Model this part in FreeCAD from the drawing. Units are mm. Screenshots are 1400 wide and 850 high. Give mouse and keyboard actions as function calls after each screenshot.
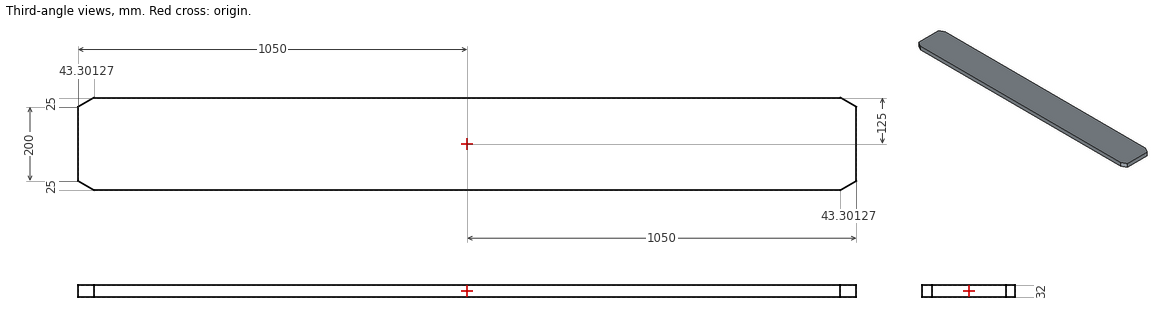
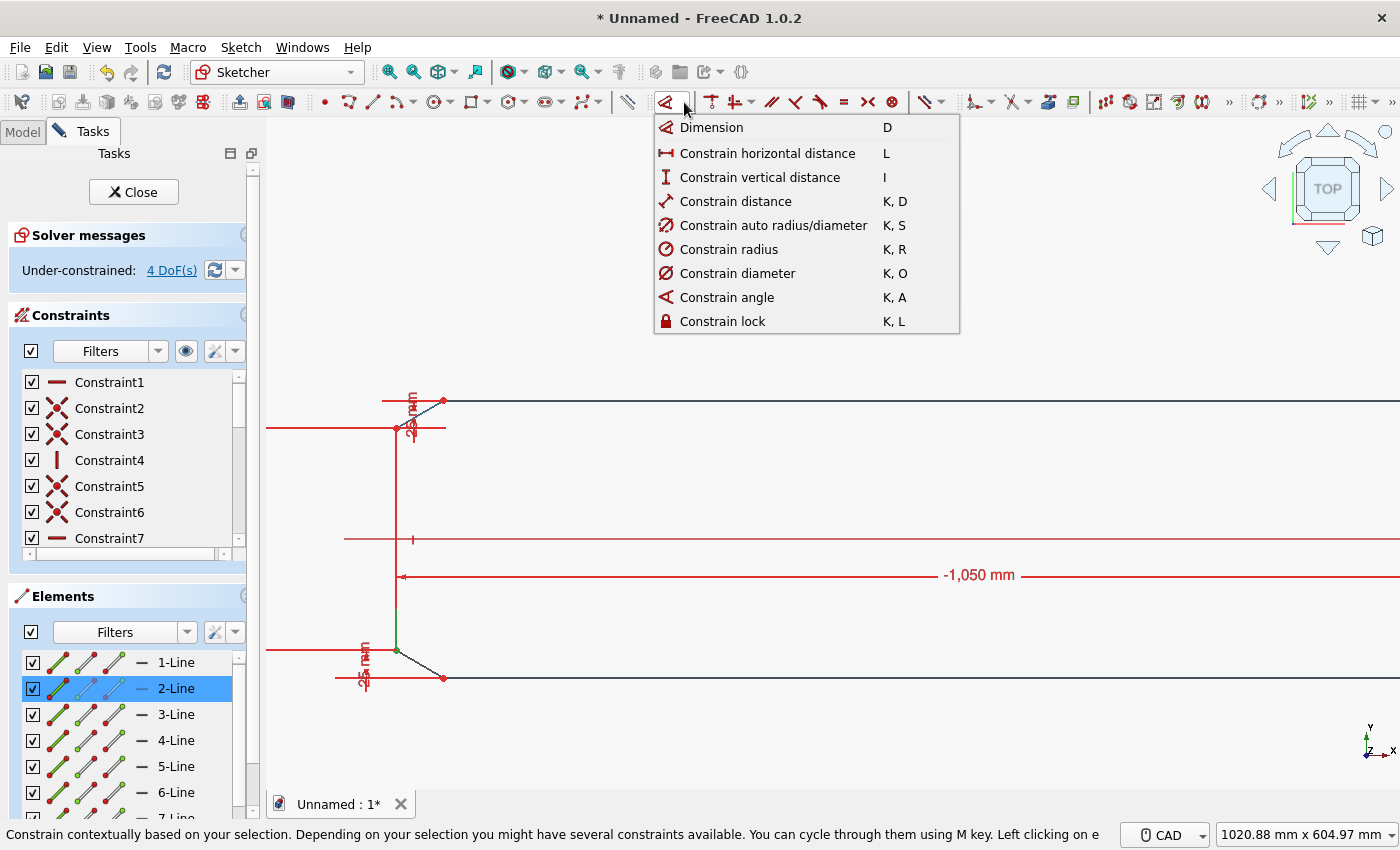
click(807, 153)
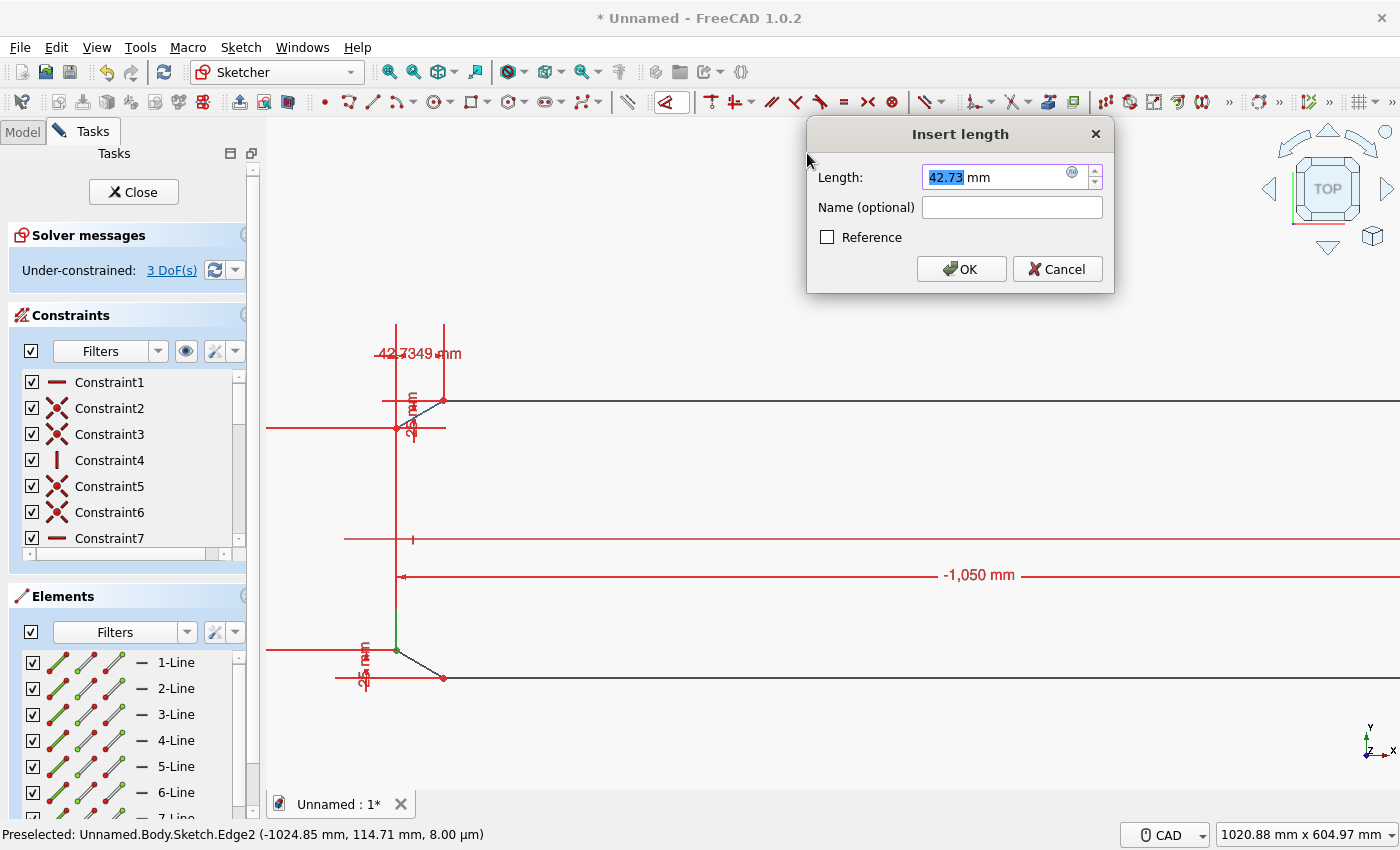
text(43.30127)
key(Return)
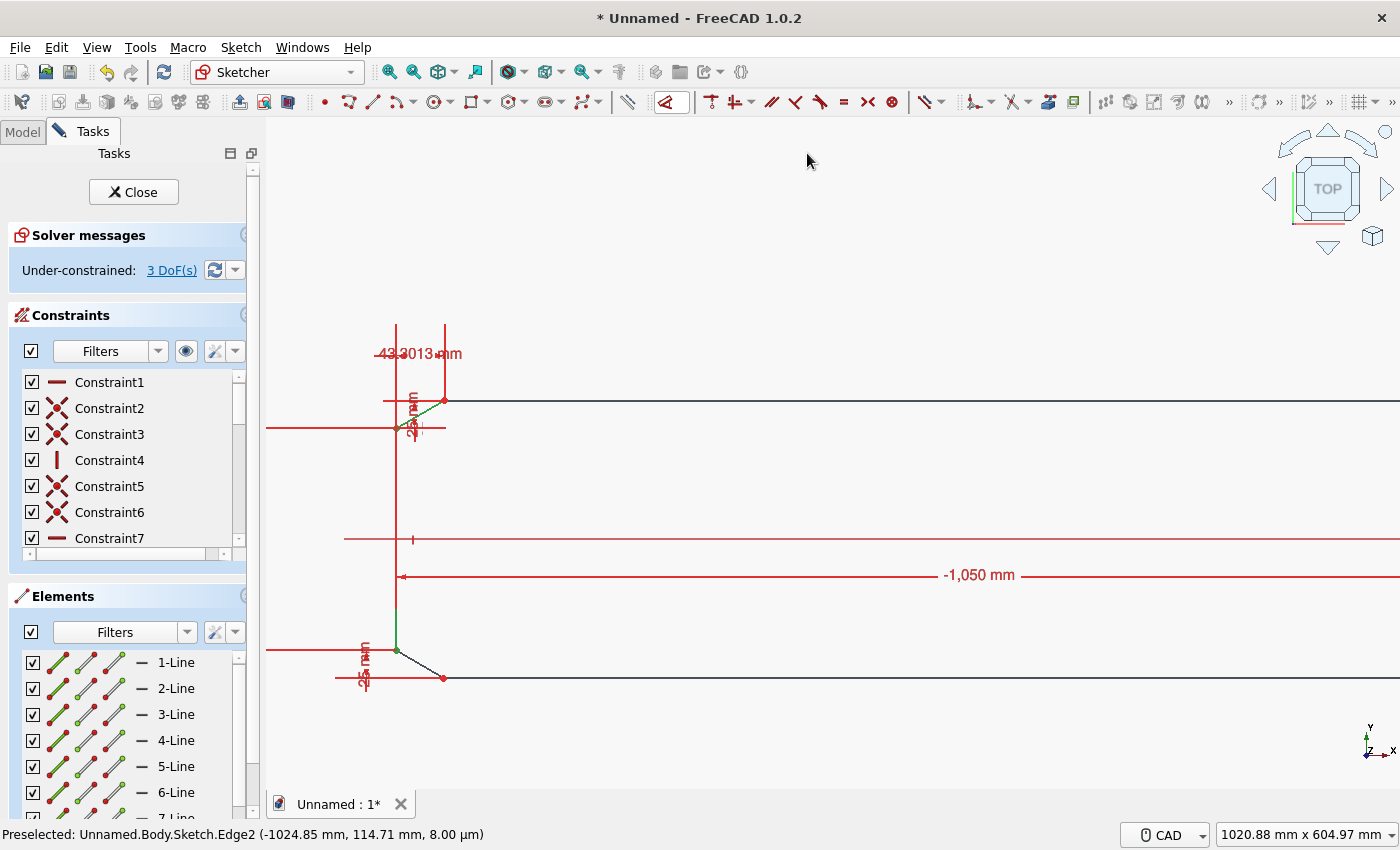
click(411, 659)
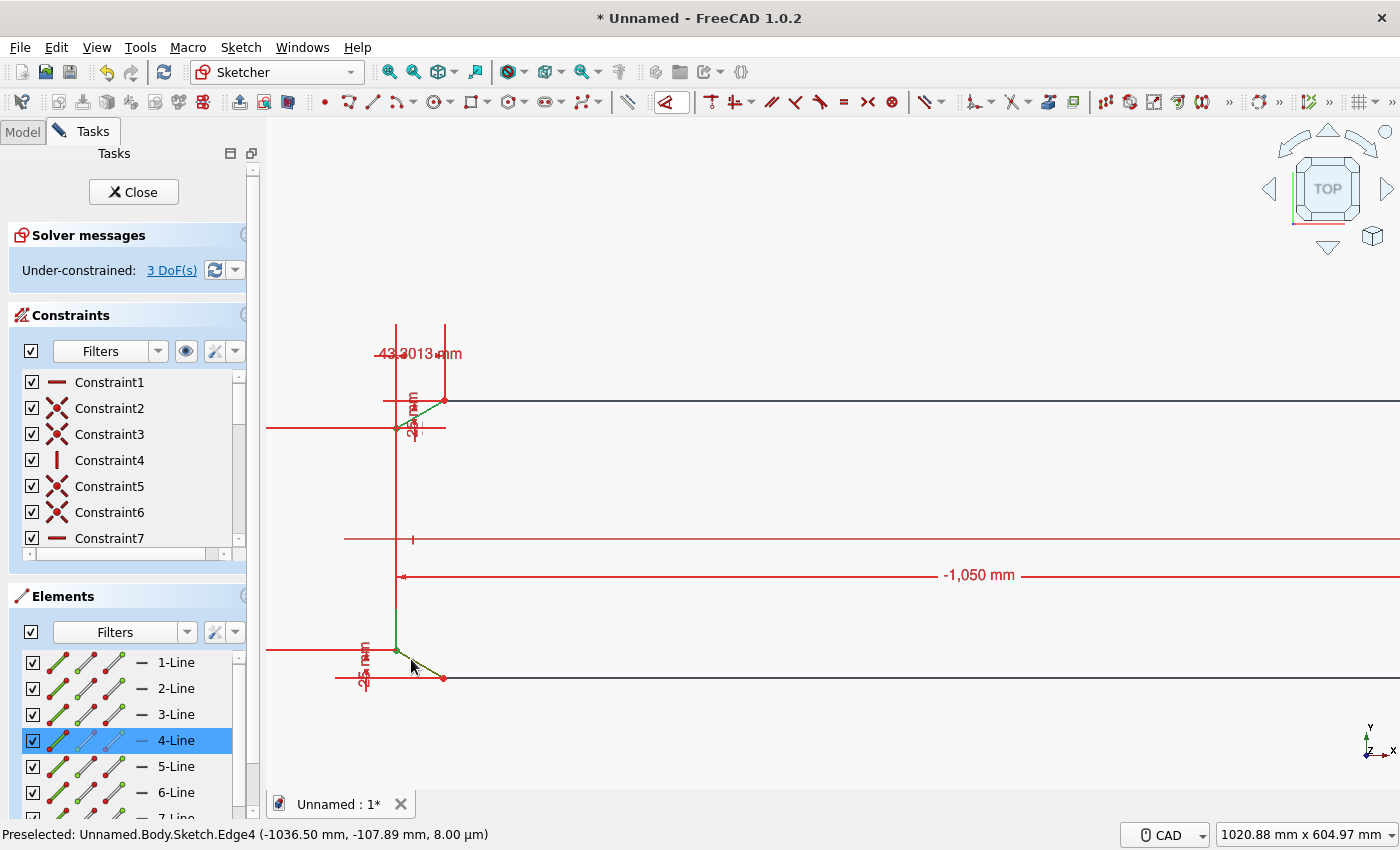
click(684, 102)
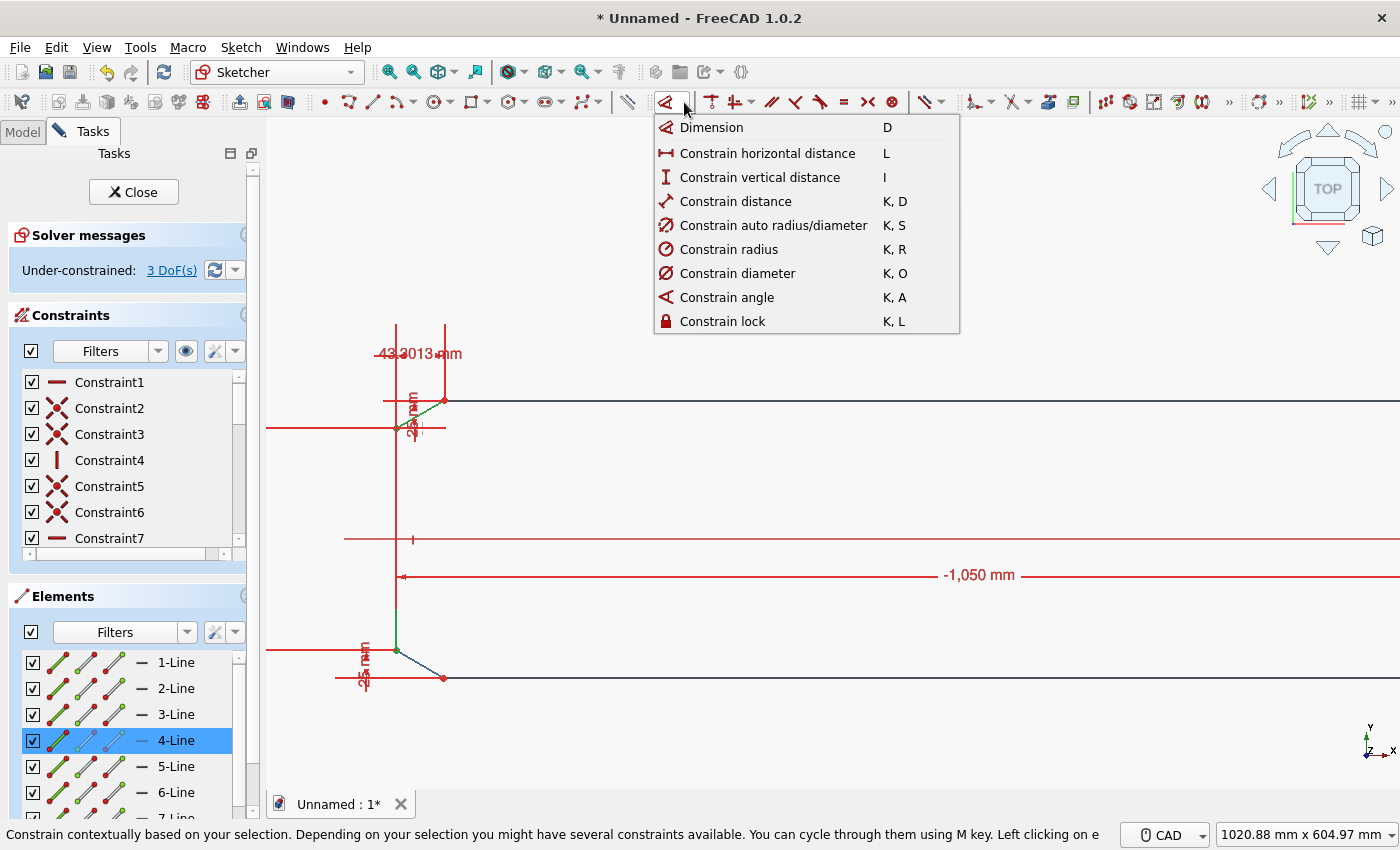
click(807, 153)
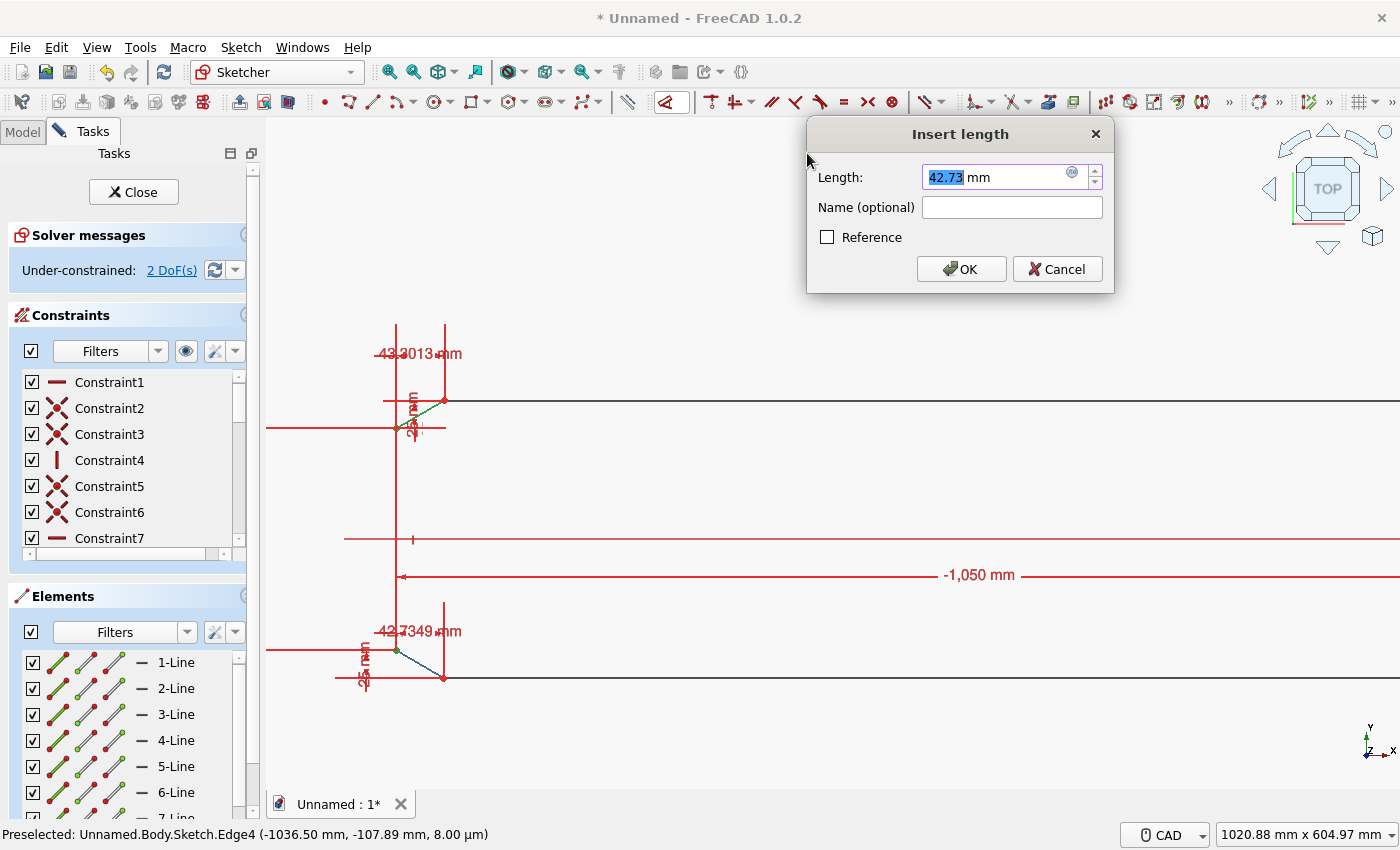
text(43.30127)
key(Return)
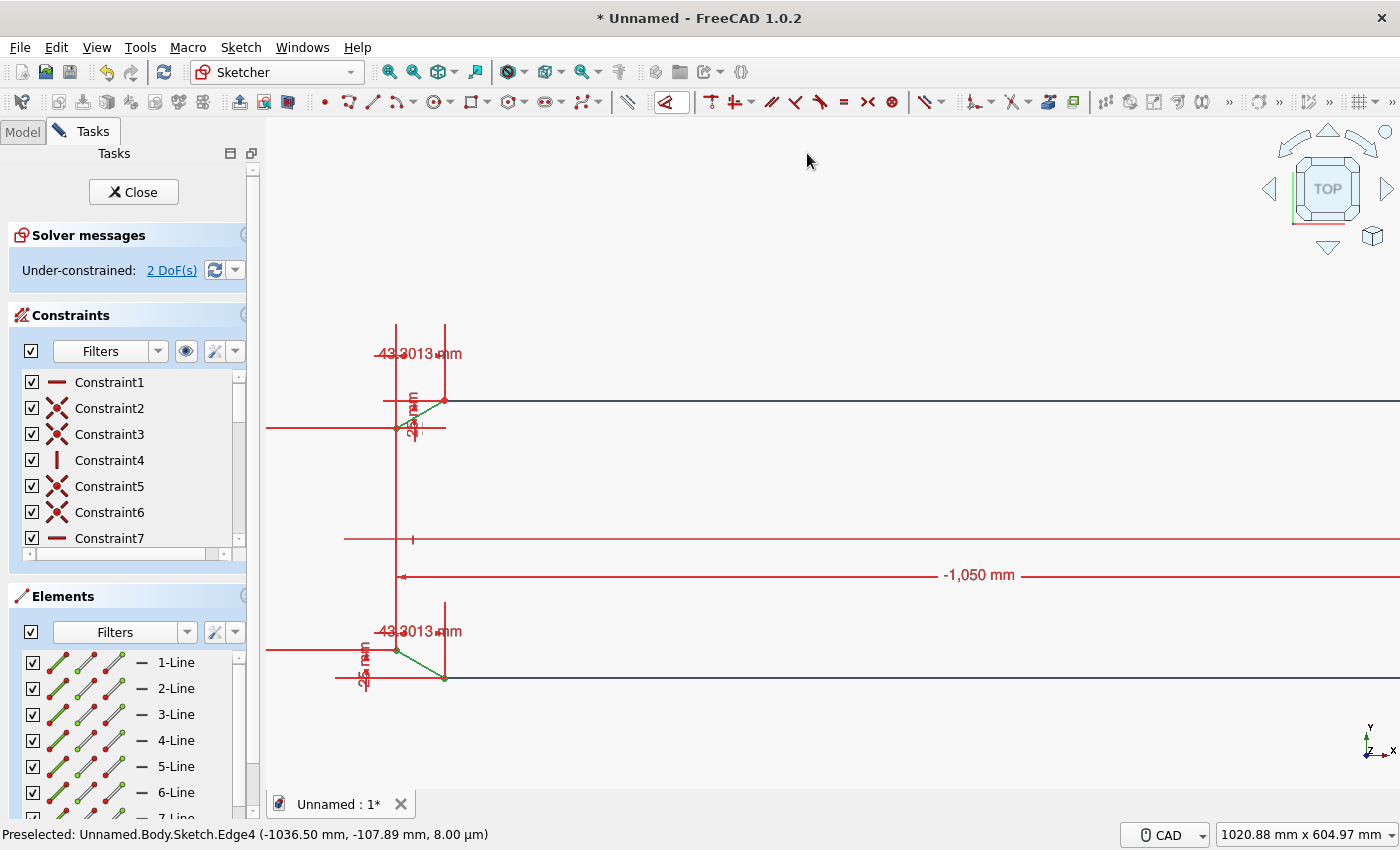
scroll(420, 416, down, 6)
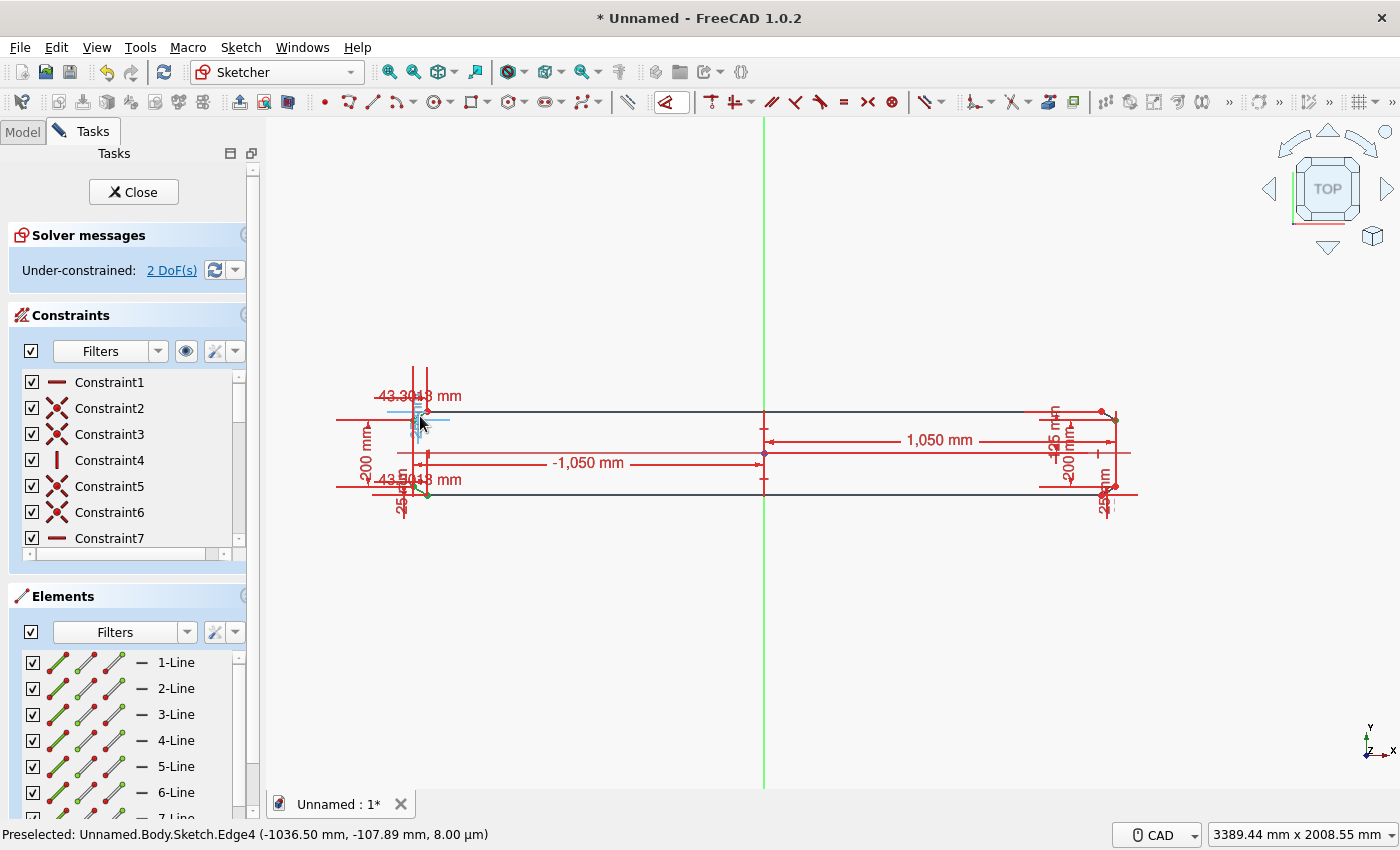
scroll(1106, 493, up, 6)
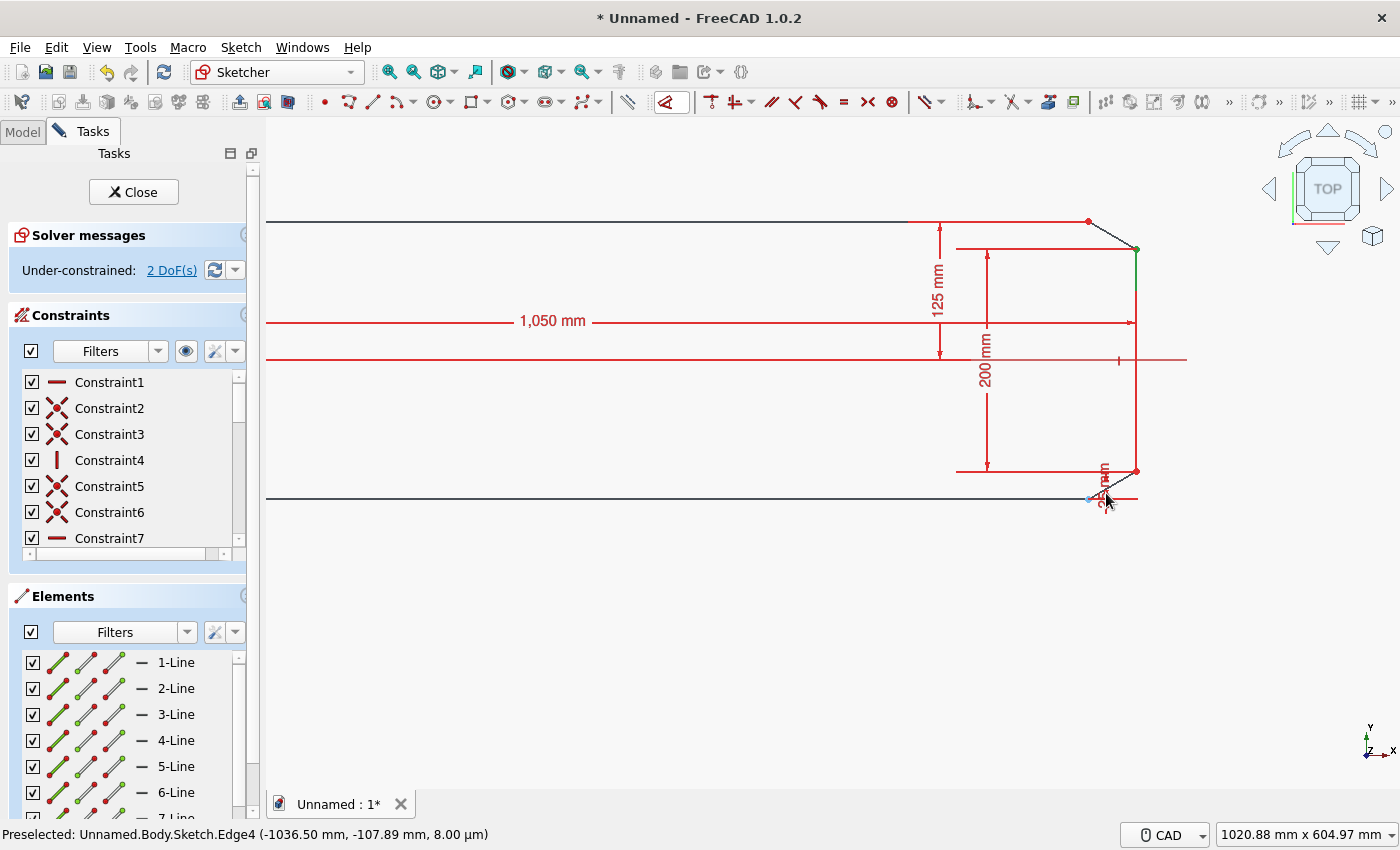
click(1122, 480)